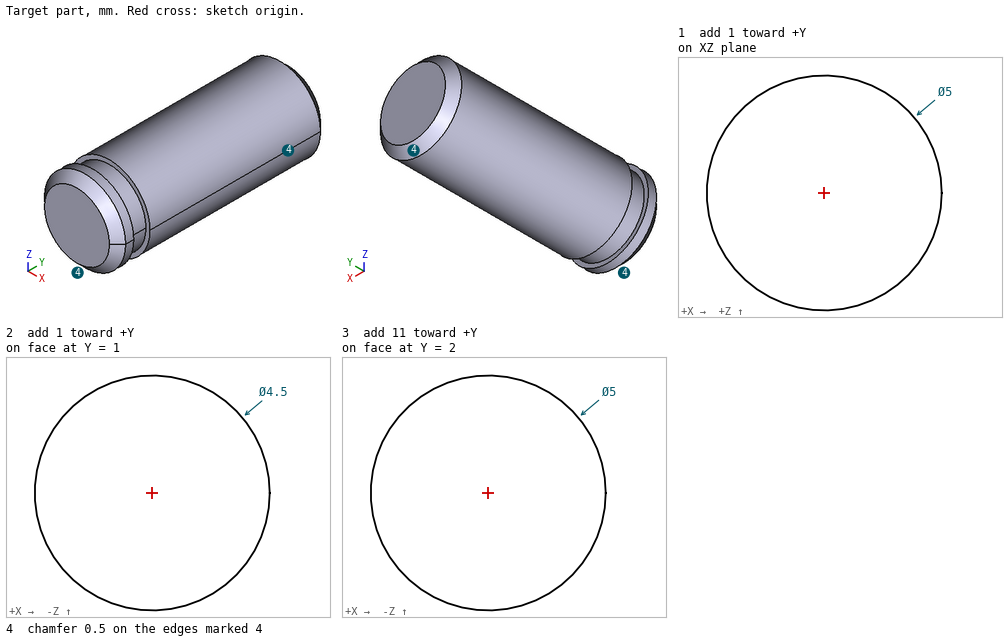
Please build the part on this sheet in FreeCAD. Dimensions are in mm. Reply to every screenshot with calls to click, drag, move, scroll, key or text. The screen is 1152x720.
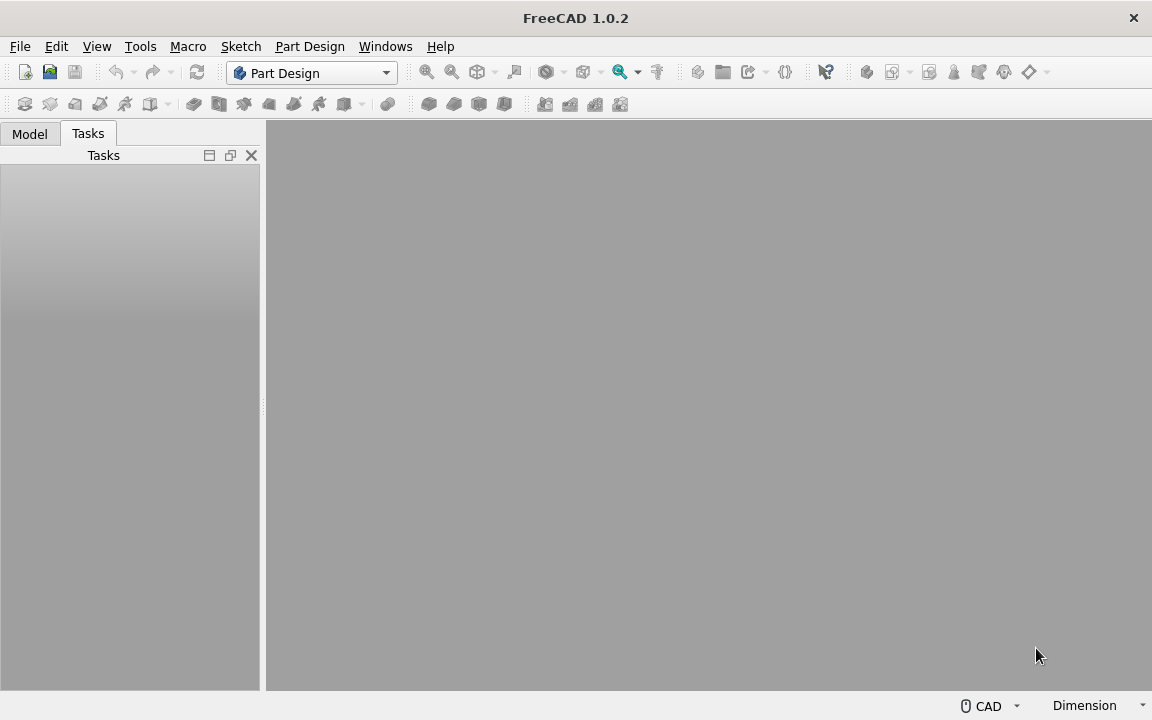
key(ctrl+n)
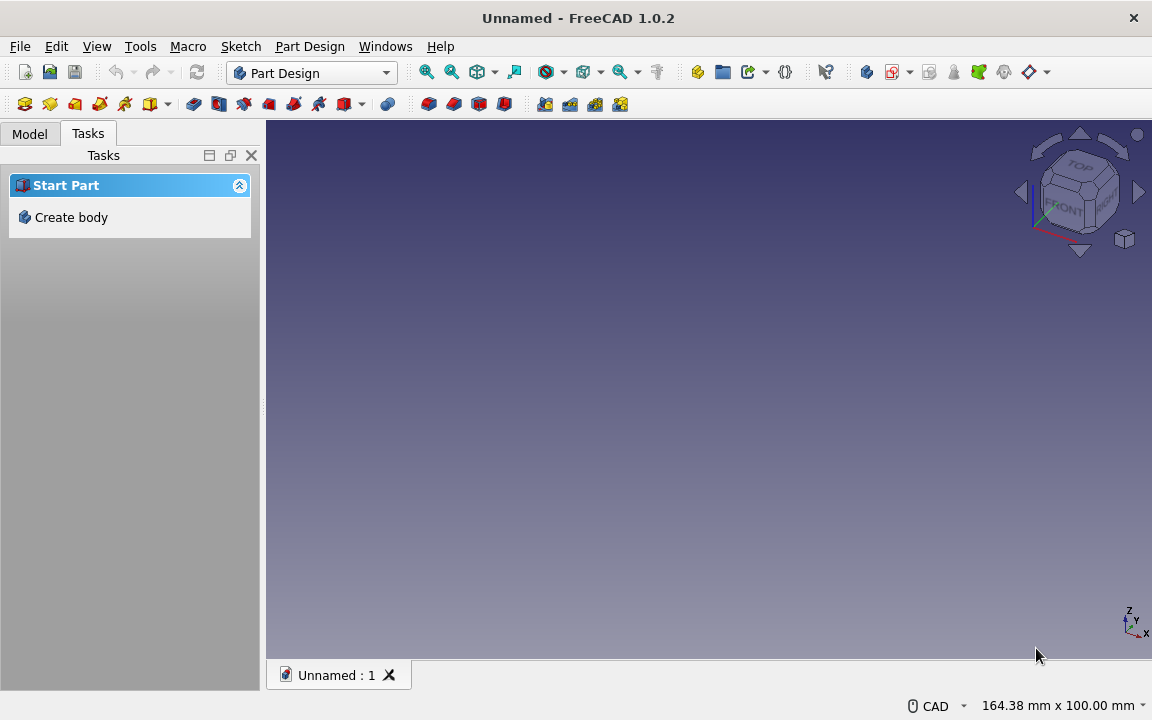
click(892, 72)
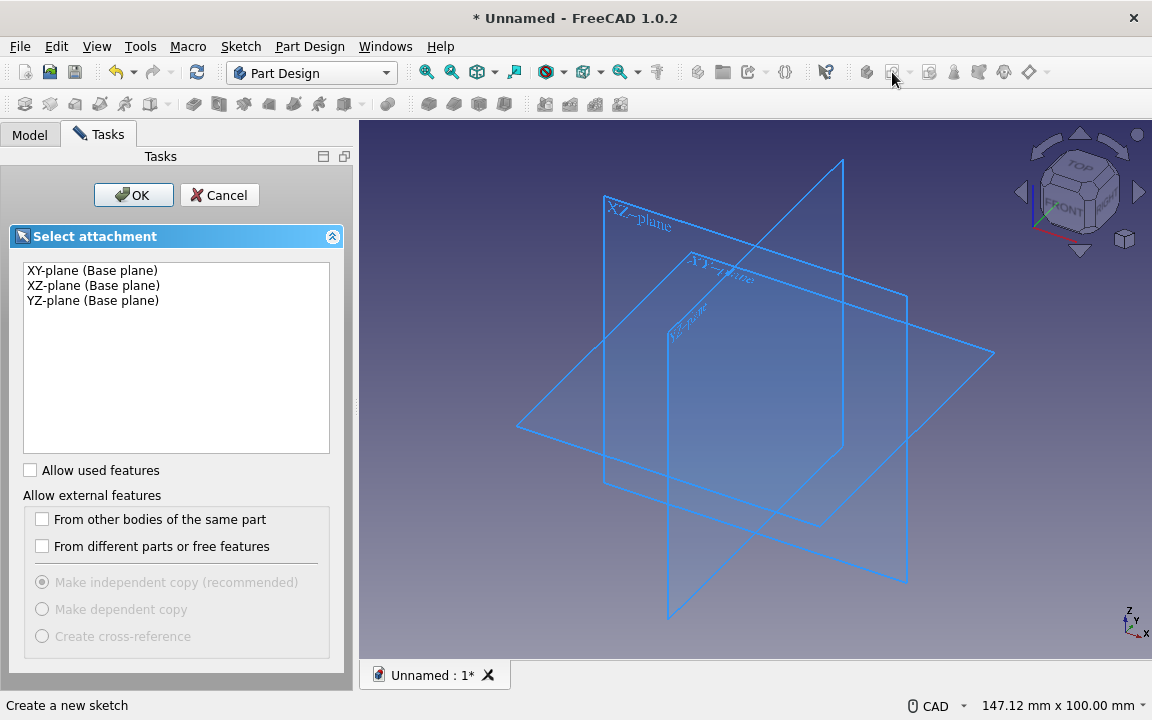
click(84, 286)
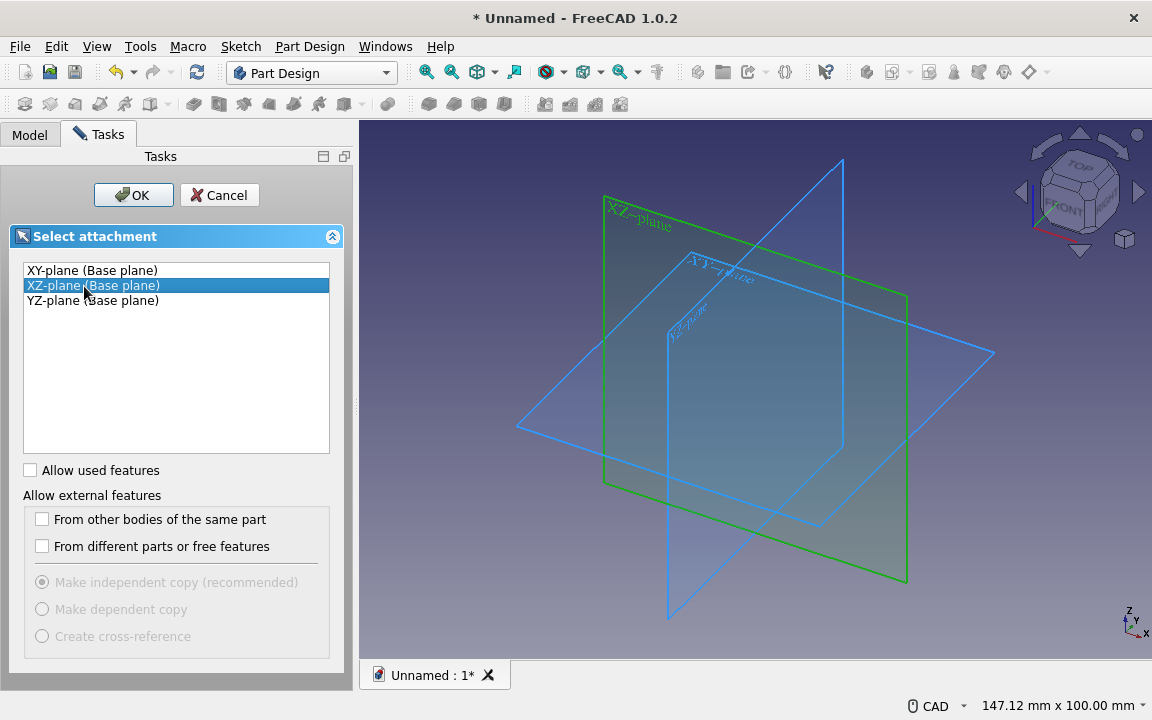
click(134, 195)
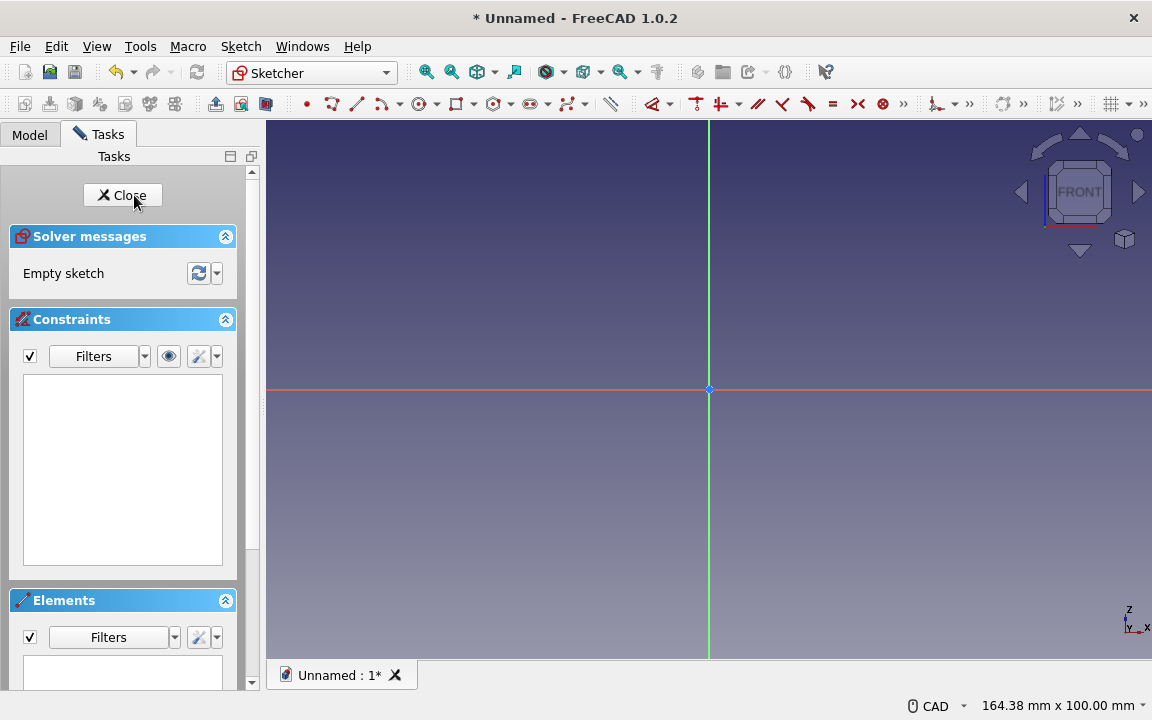
scroll(714, 390, up, 13)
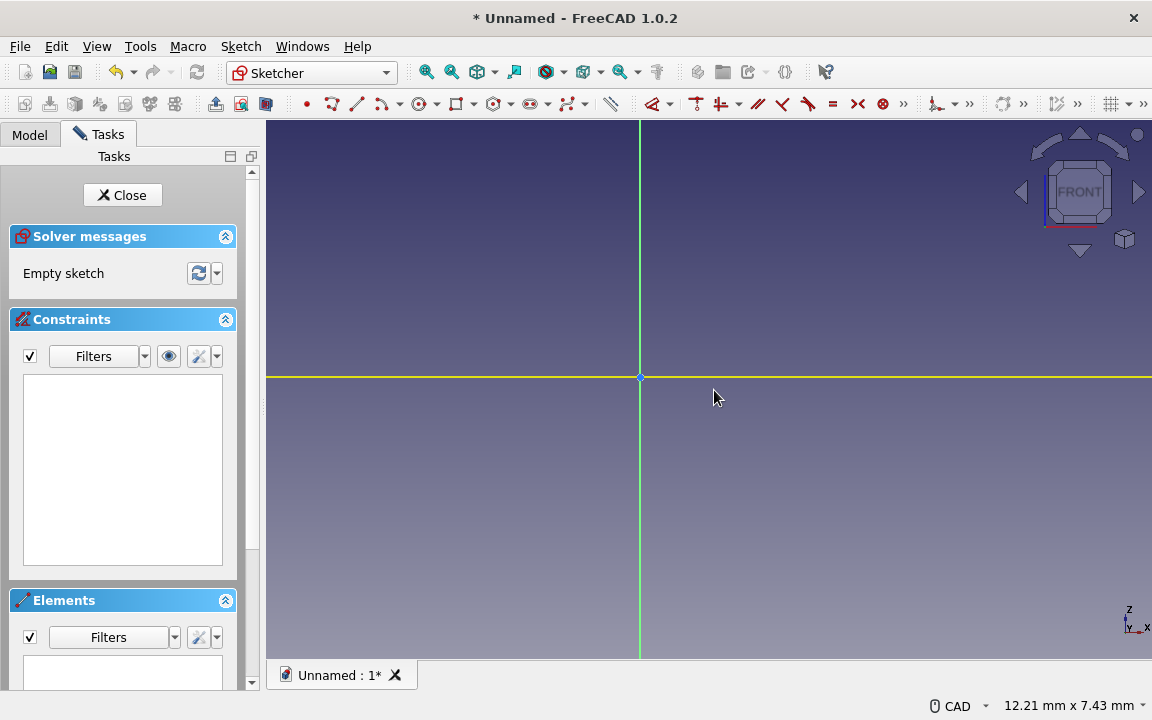
click(418, 104)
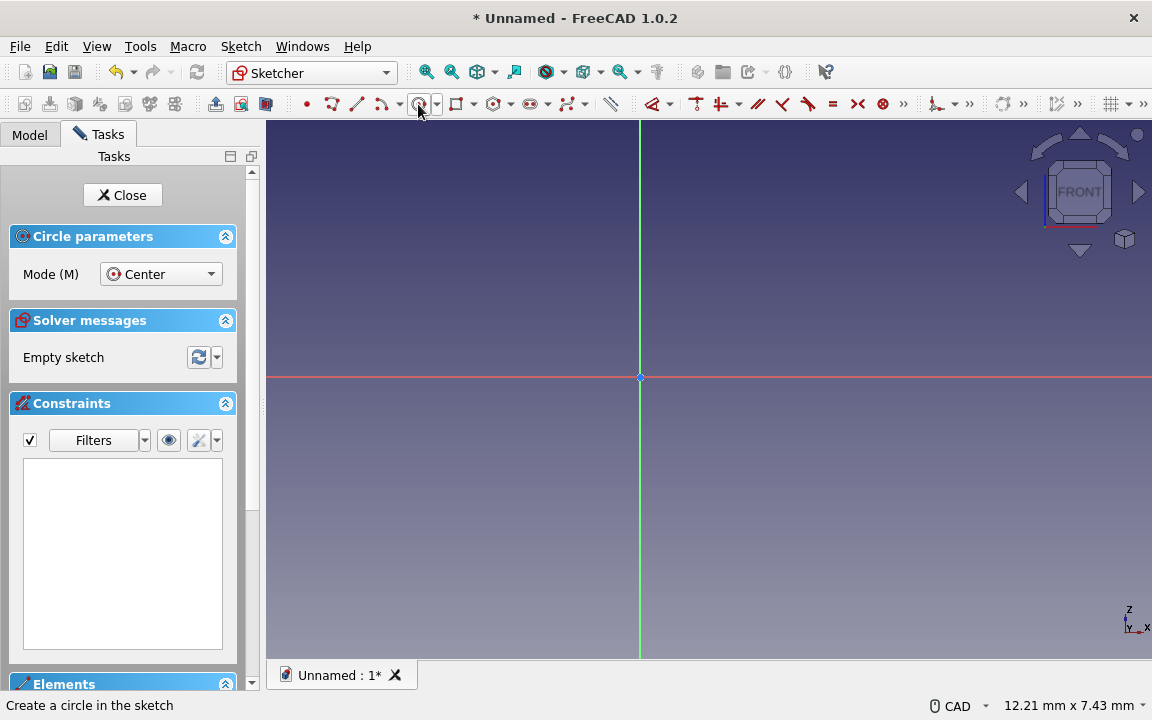
click(640, 377)
click(769, 249)
key(Escape)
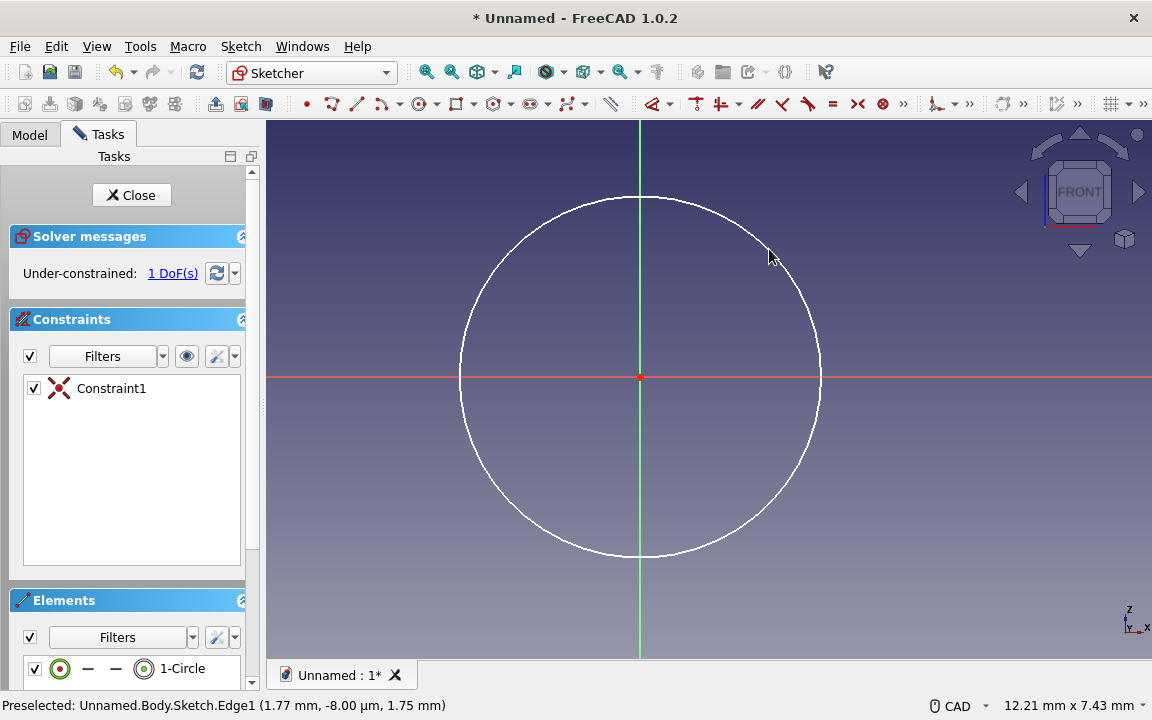
key(d)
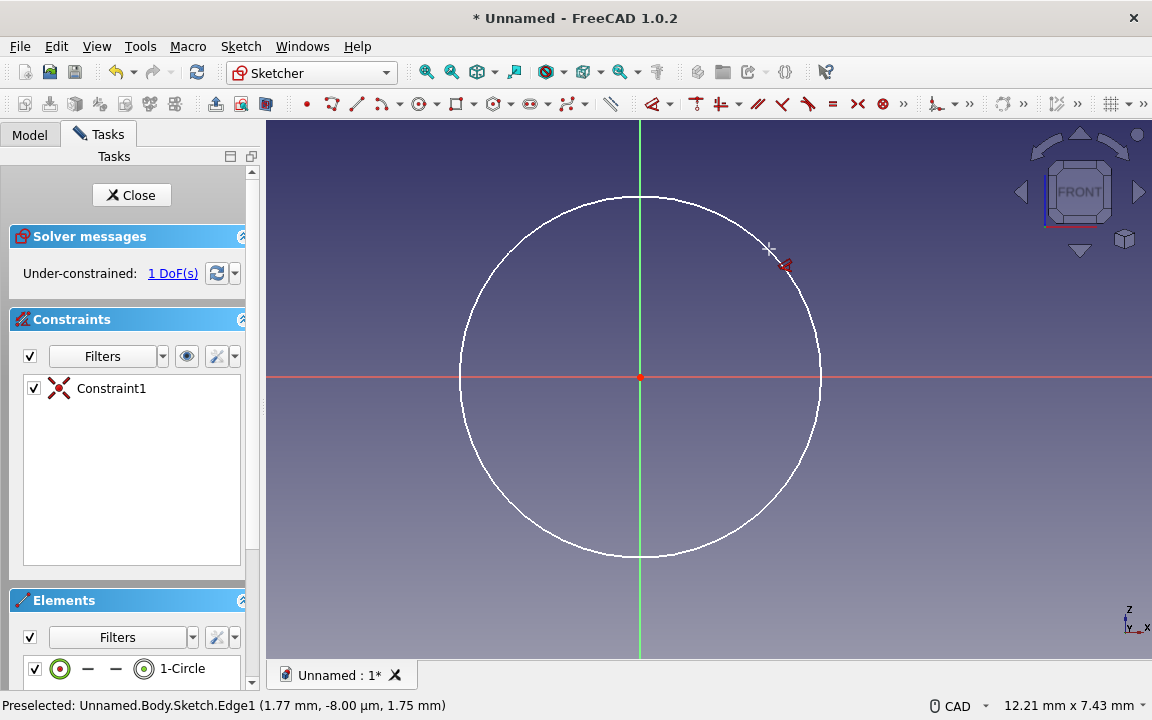
click(768, 249)
click(791, 226)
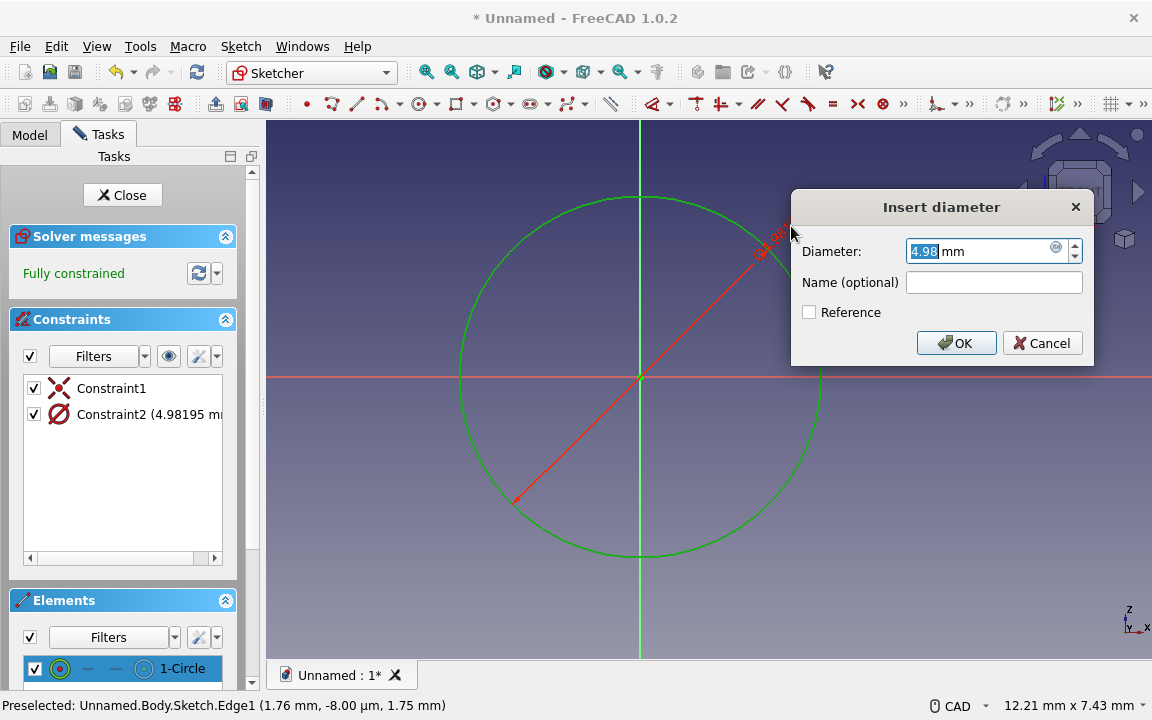
text(5)
key(Return)
key(Escape)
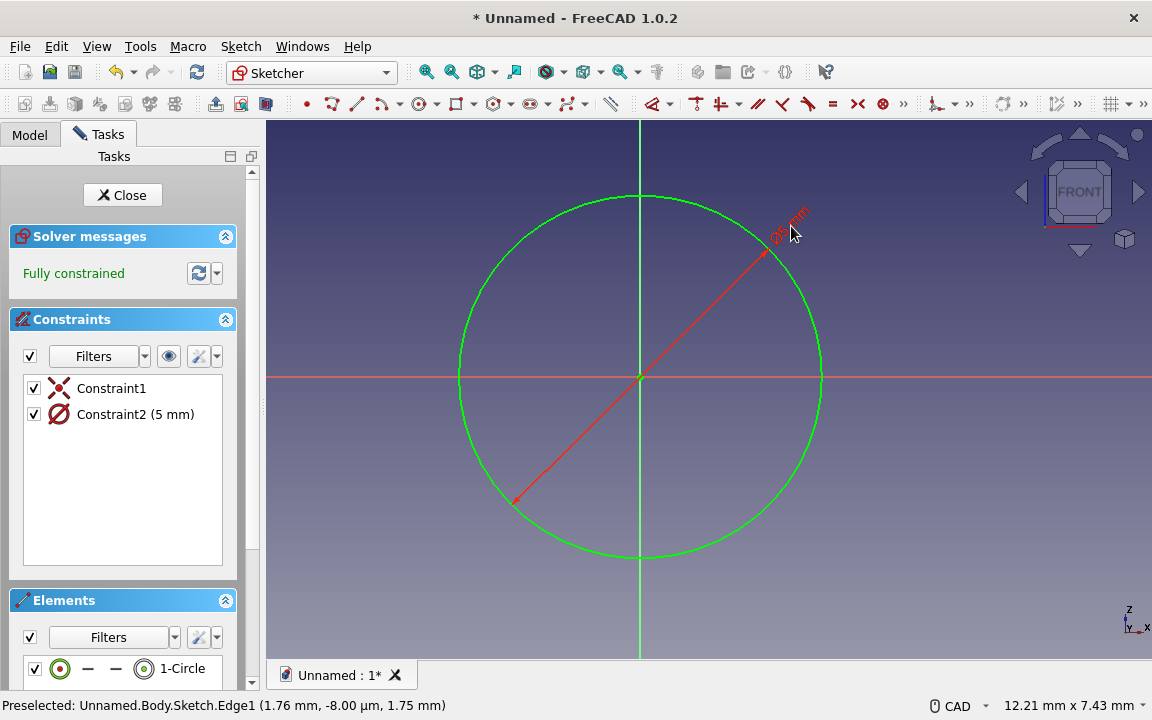
click(123, 195)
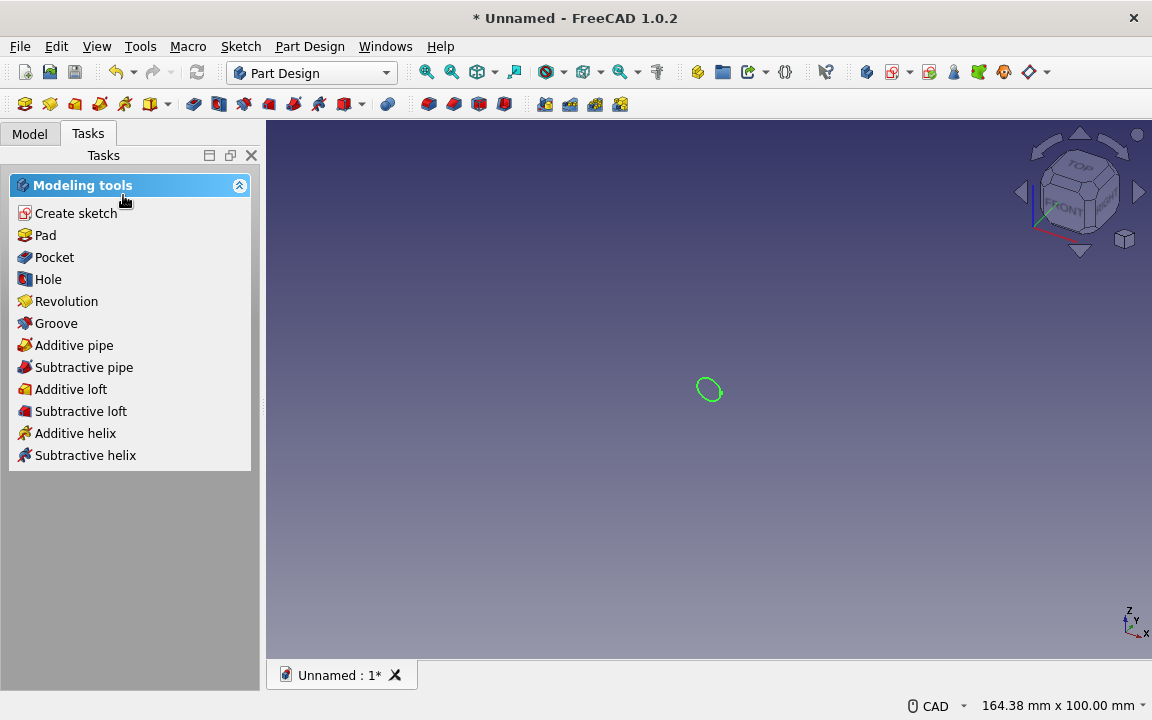
click(25, 104)